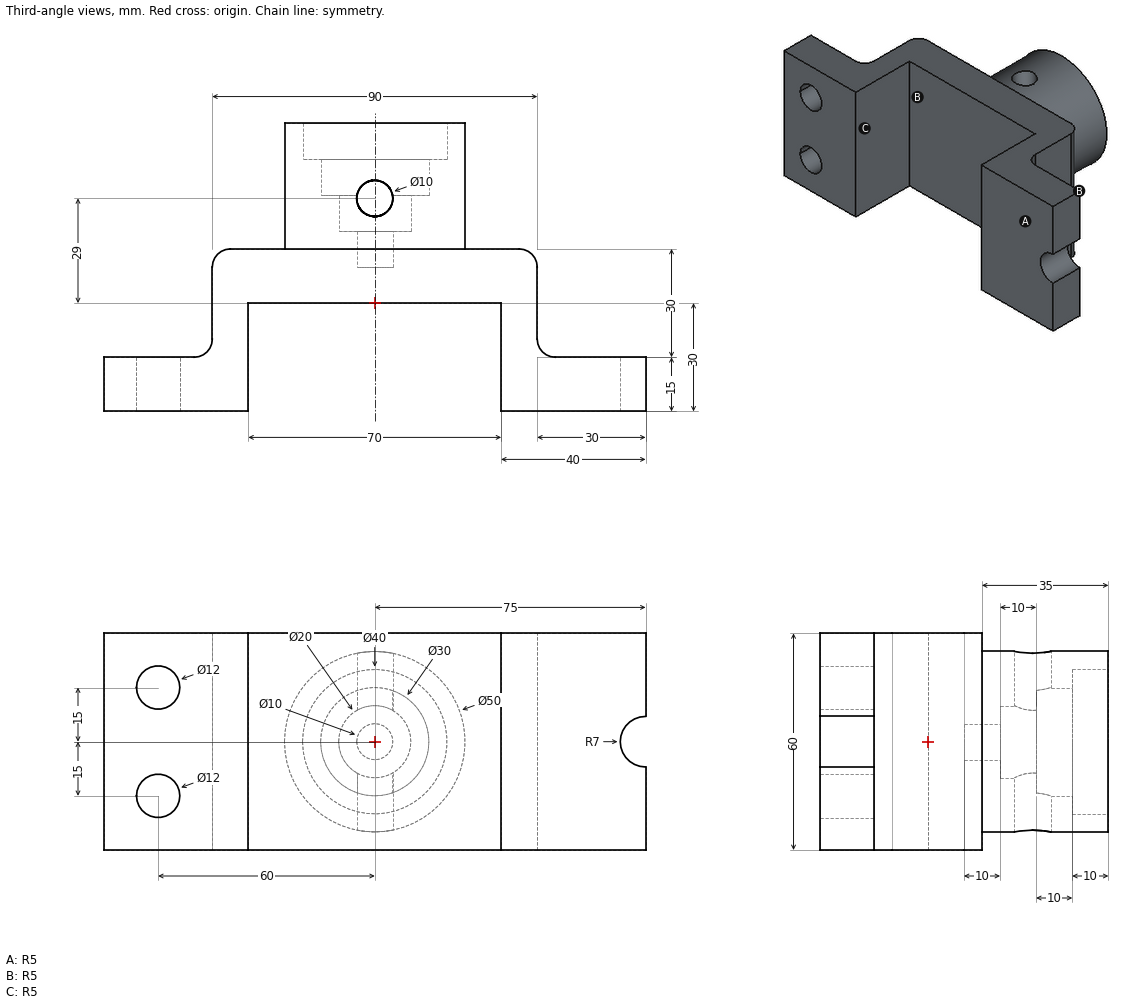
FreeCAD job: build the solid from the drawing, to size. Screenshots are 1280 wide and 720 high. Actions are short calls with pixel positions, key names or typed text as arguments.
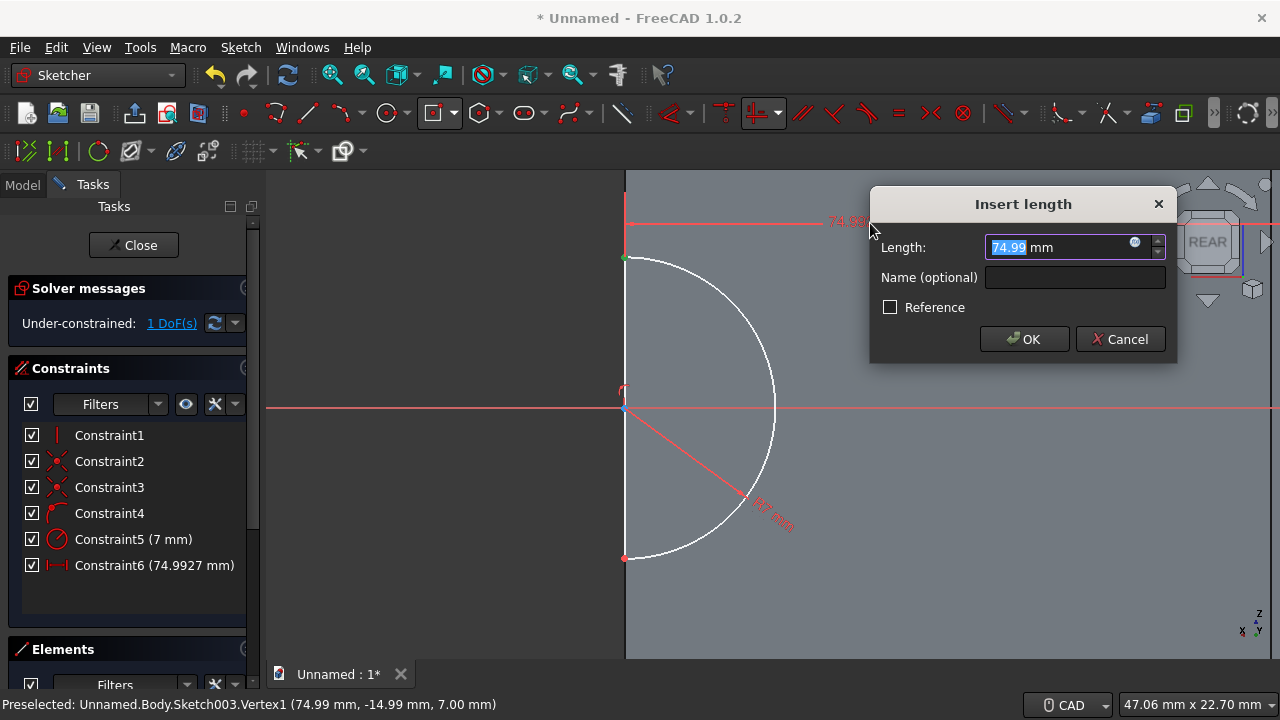
text(75)
key(Return)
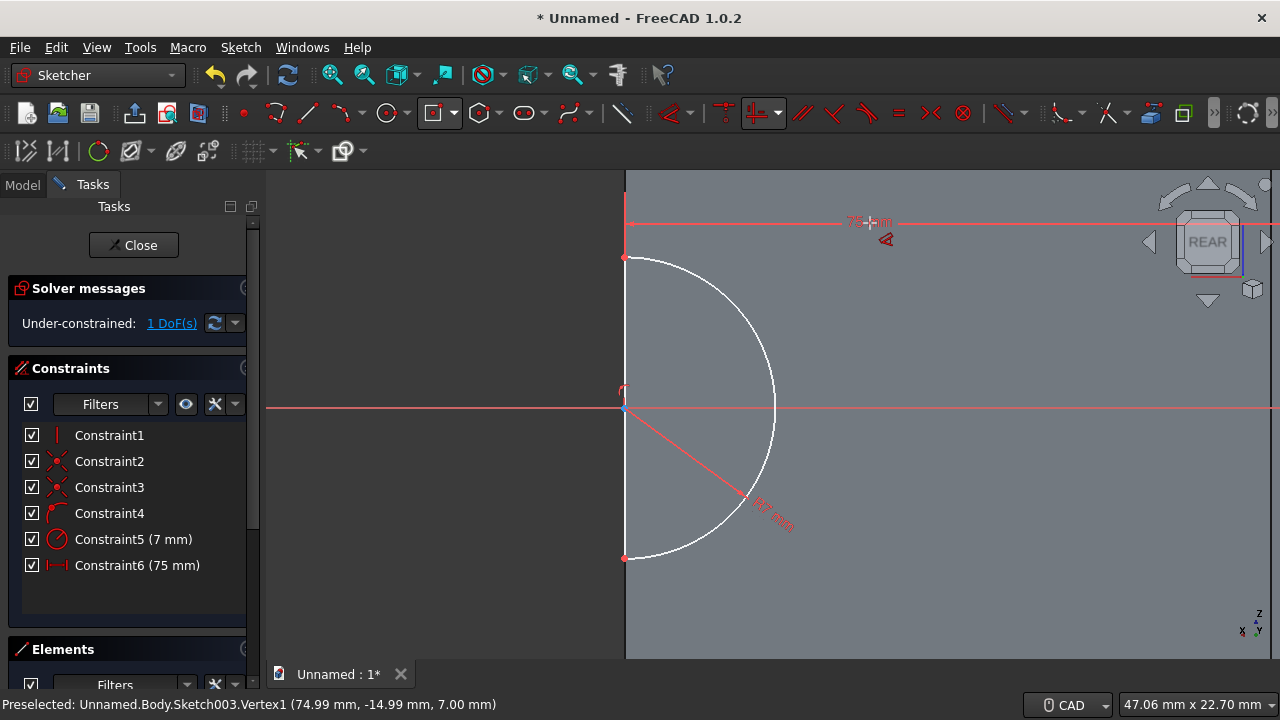
click(624, 408)
click(870, 442)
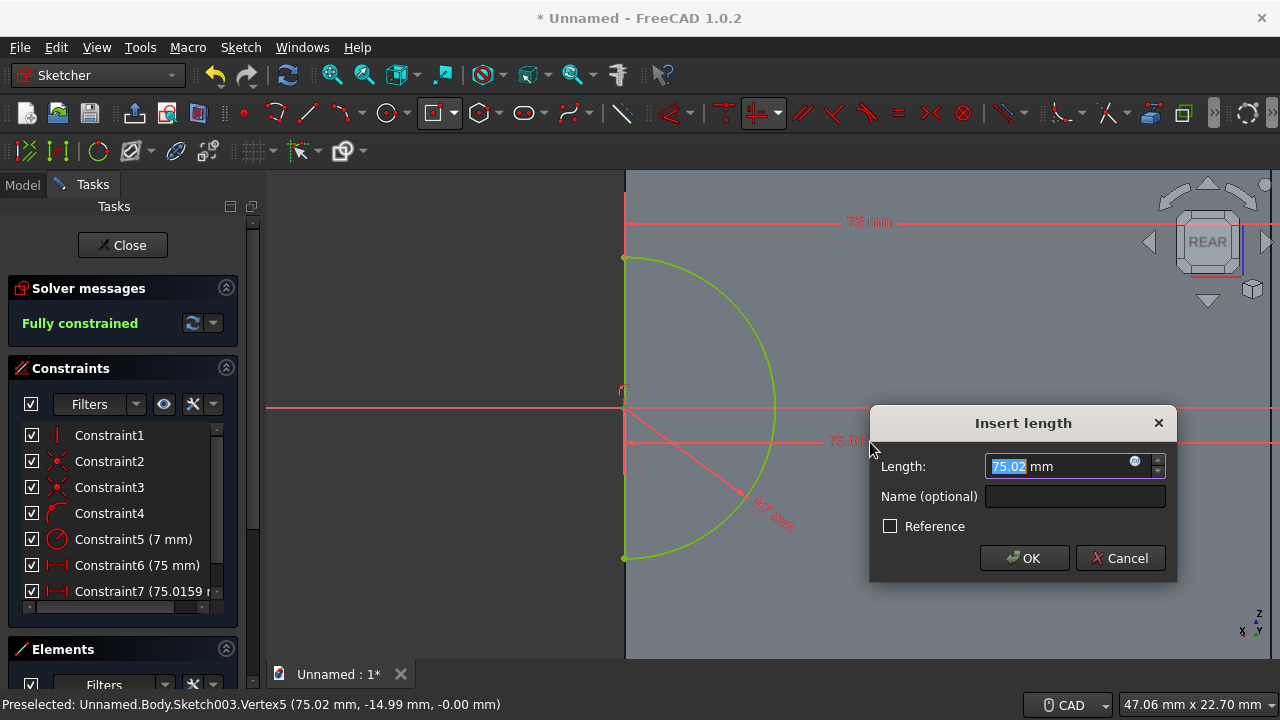
text(75)
key(Return)
key(Escape)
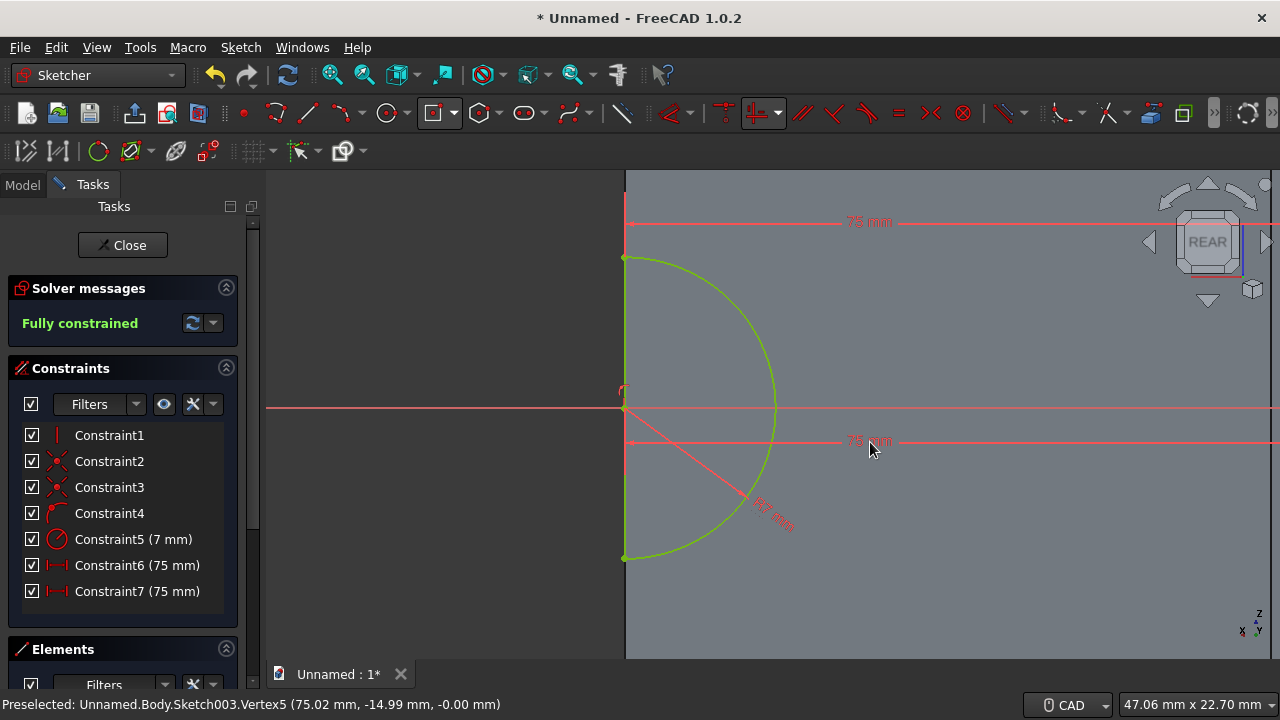
click(123, 245)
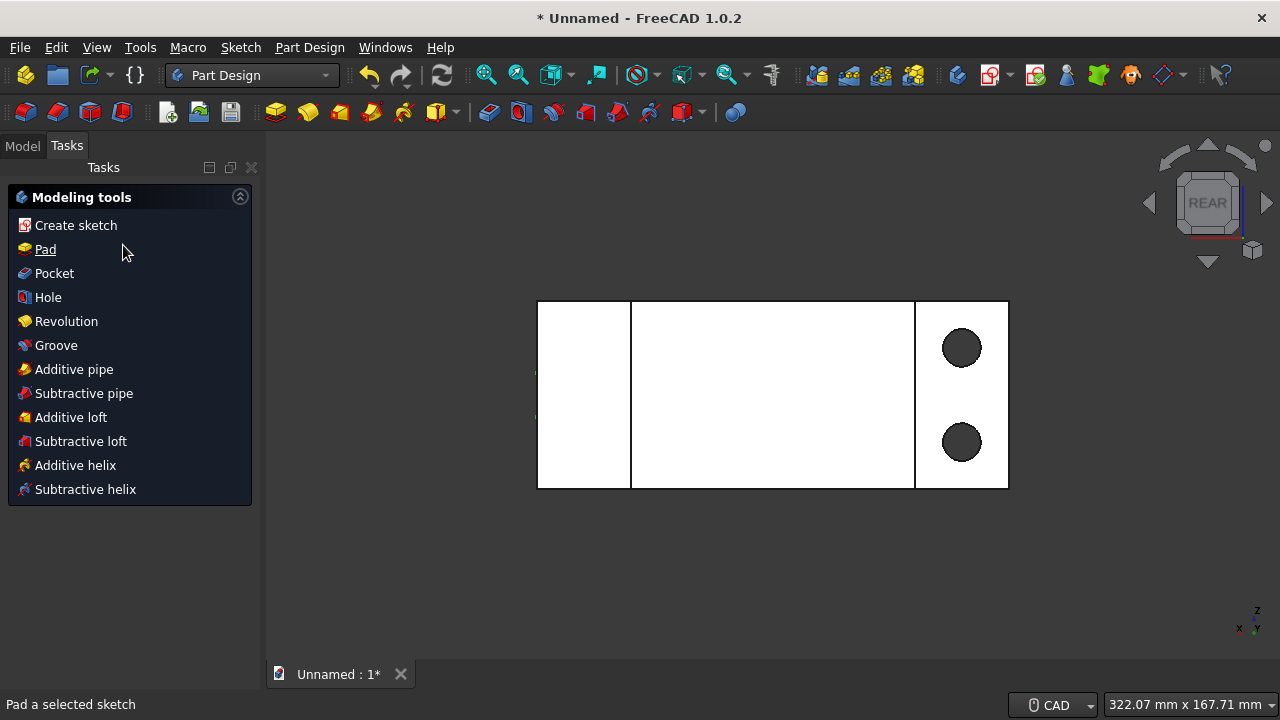
click(490, 112)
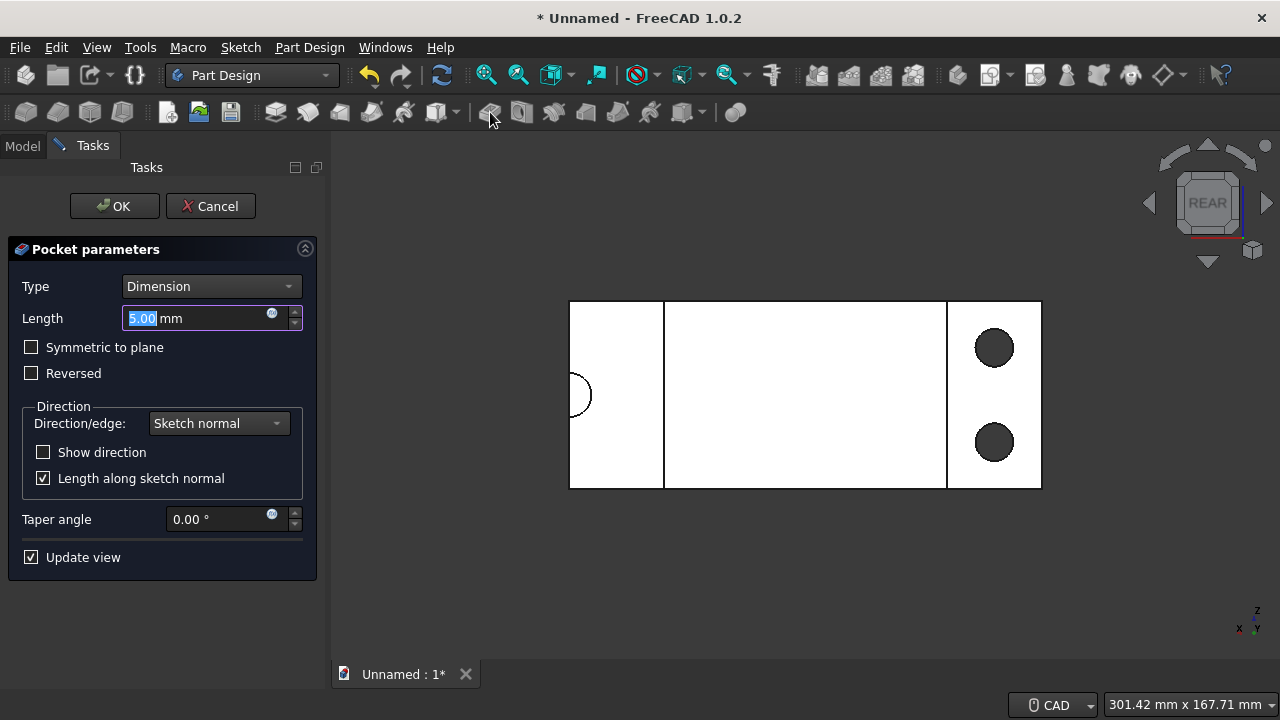
click(212, 286)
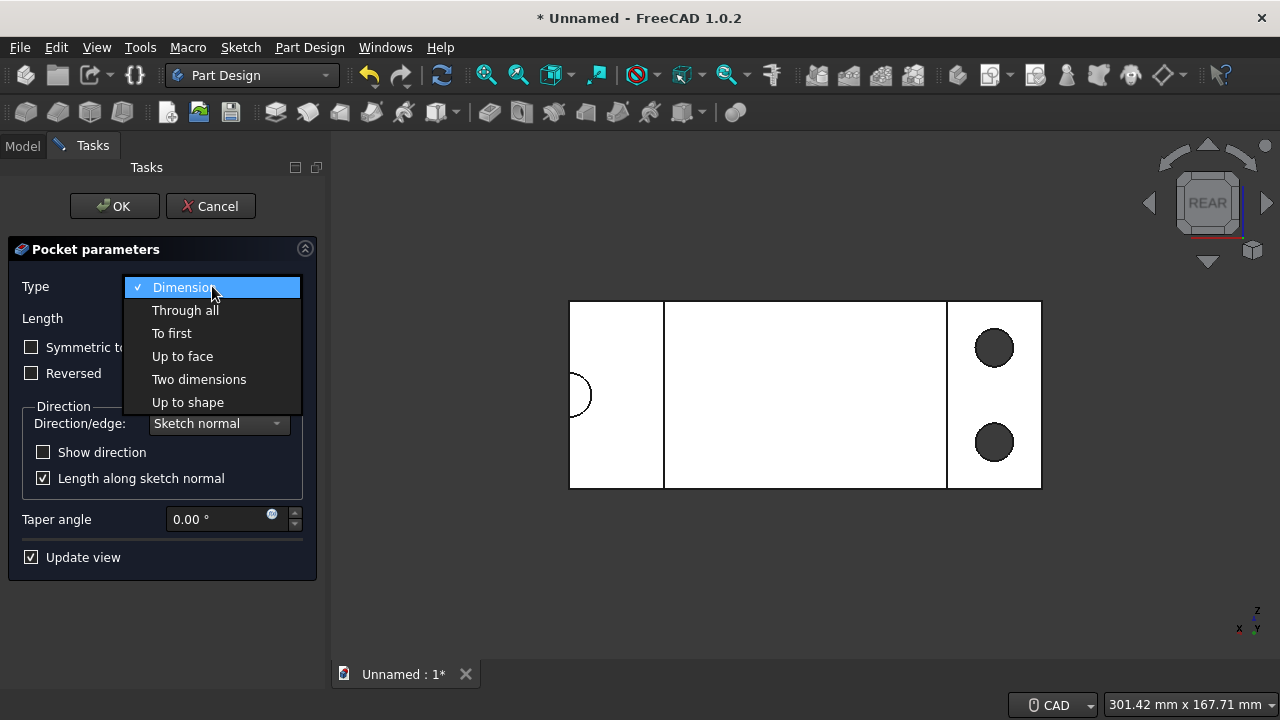
click(212, 334)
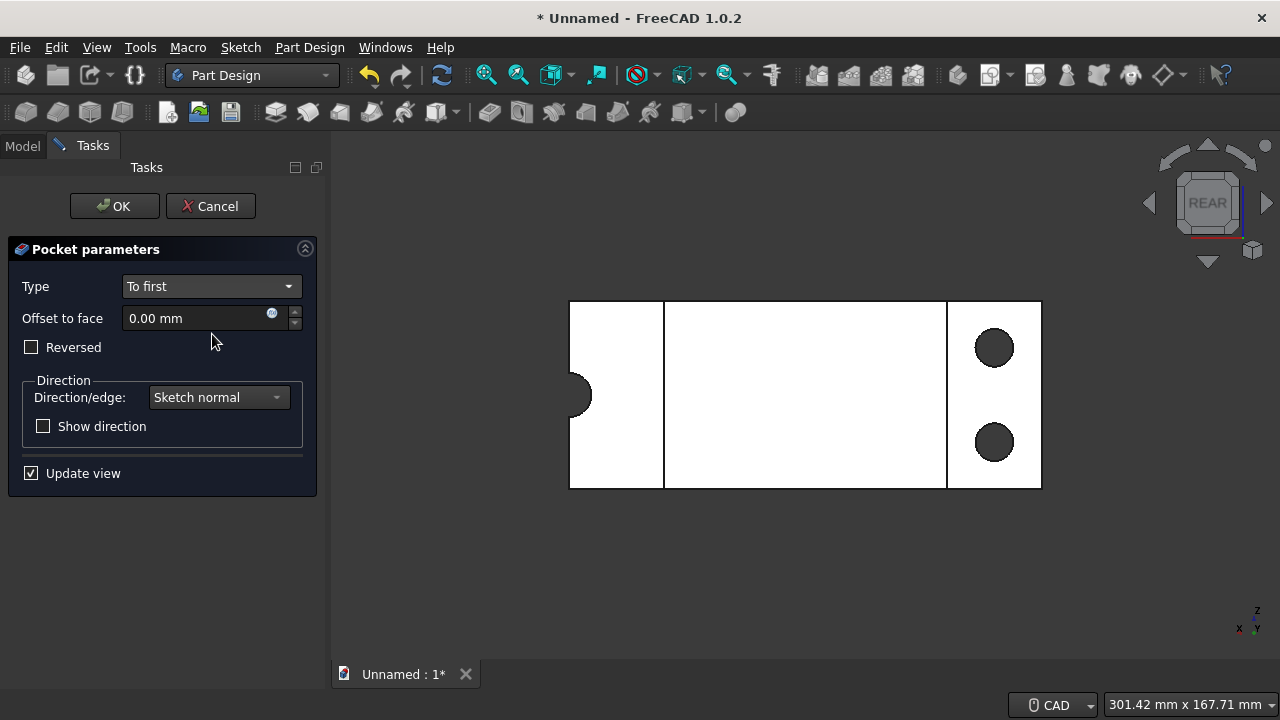
click(115, 206)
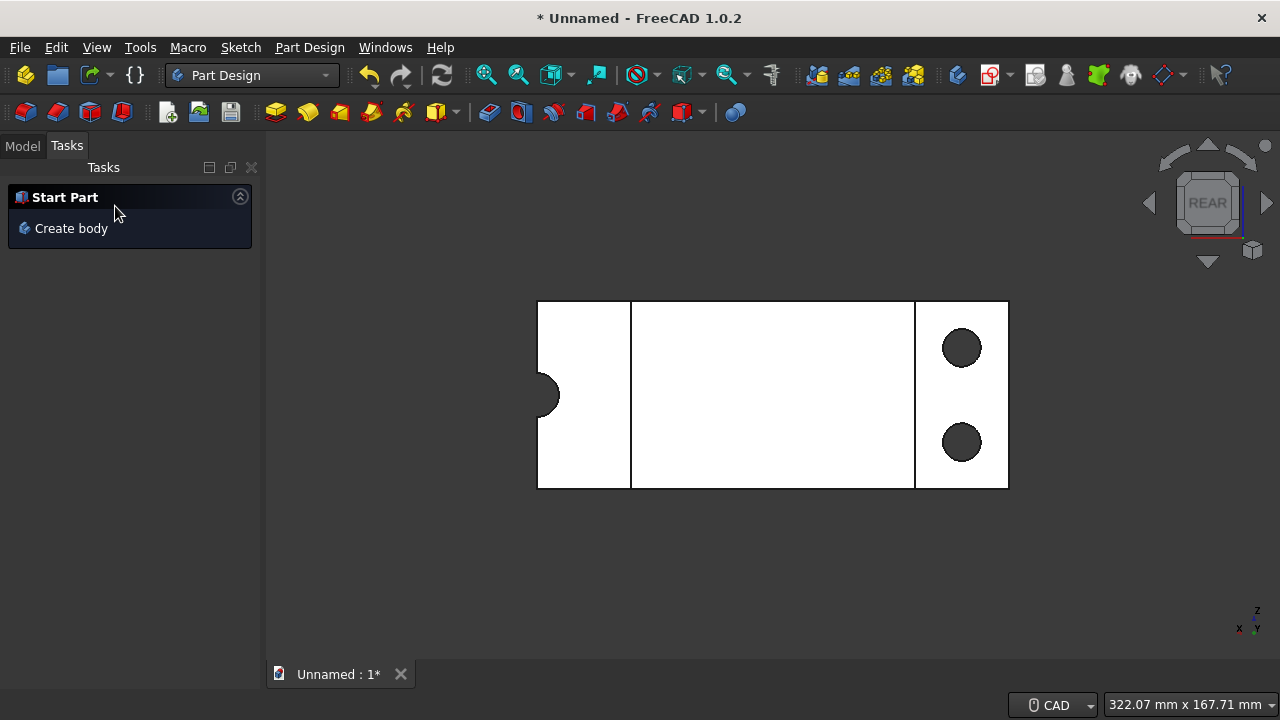
click(733, 394)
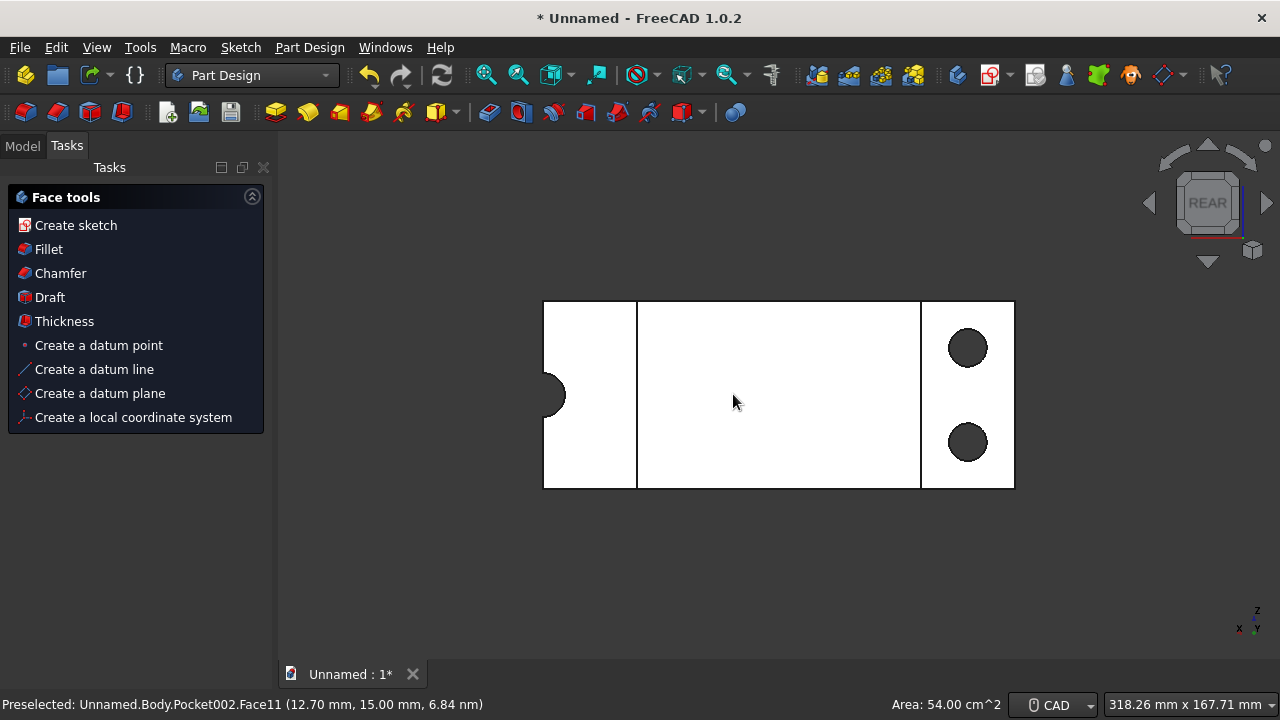
click(990, 76)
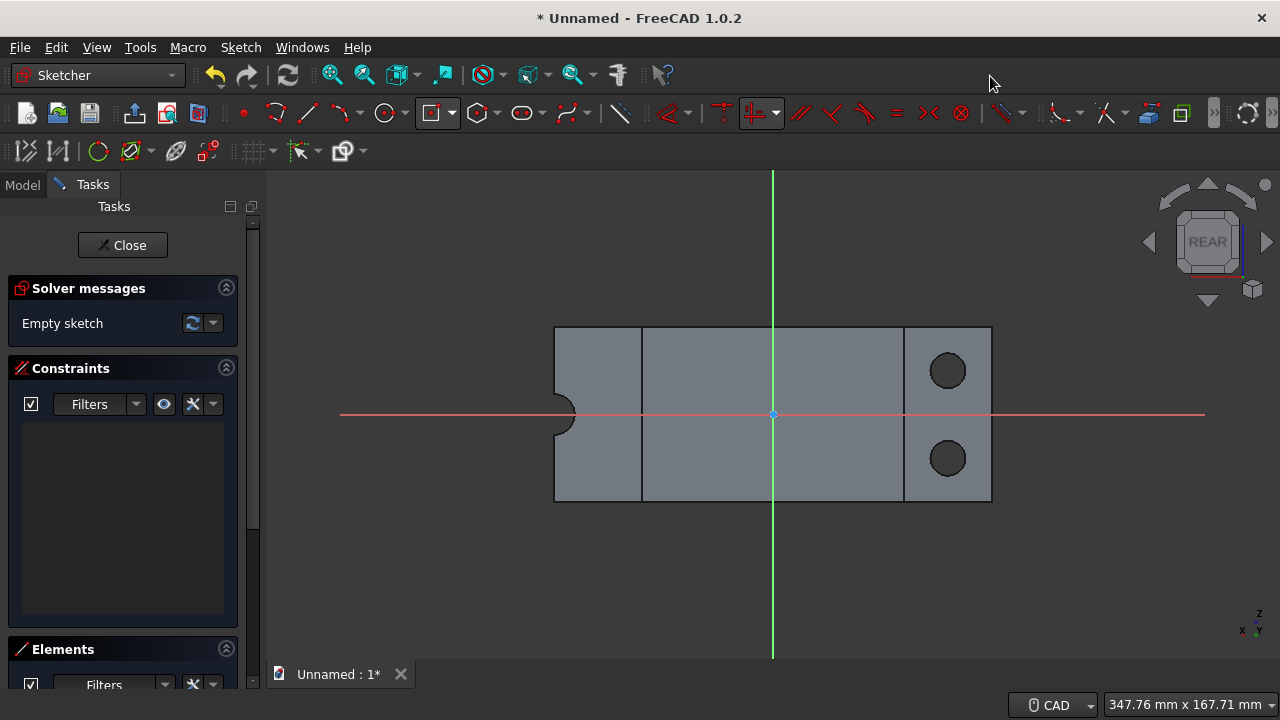
scroll(829, 415, up, 4)